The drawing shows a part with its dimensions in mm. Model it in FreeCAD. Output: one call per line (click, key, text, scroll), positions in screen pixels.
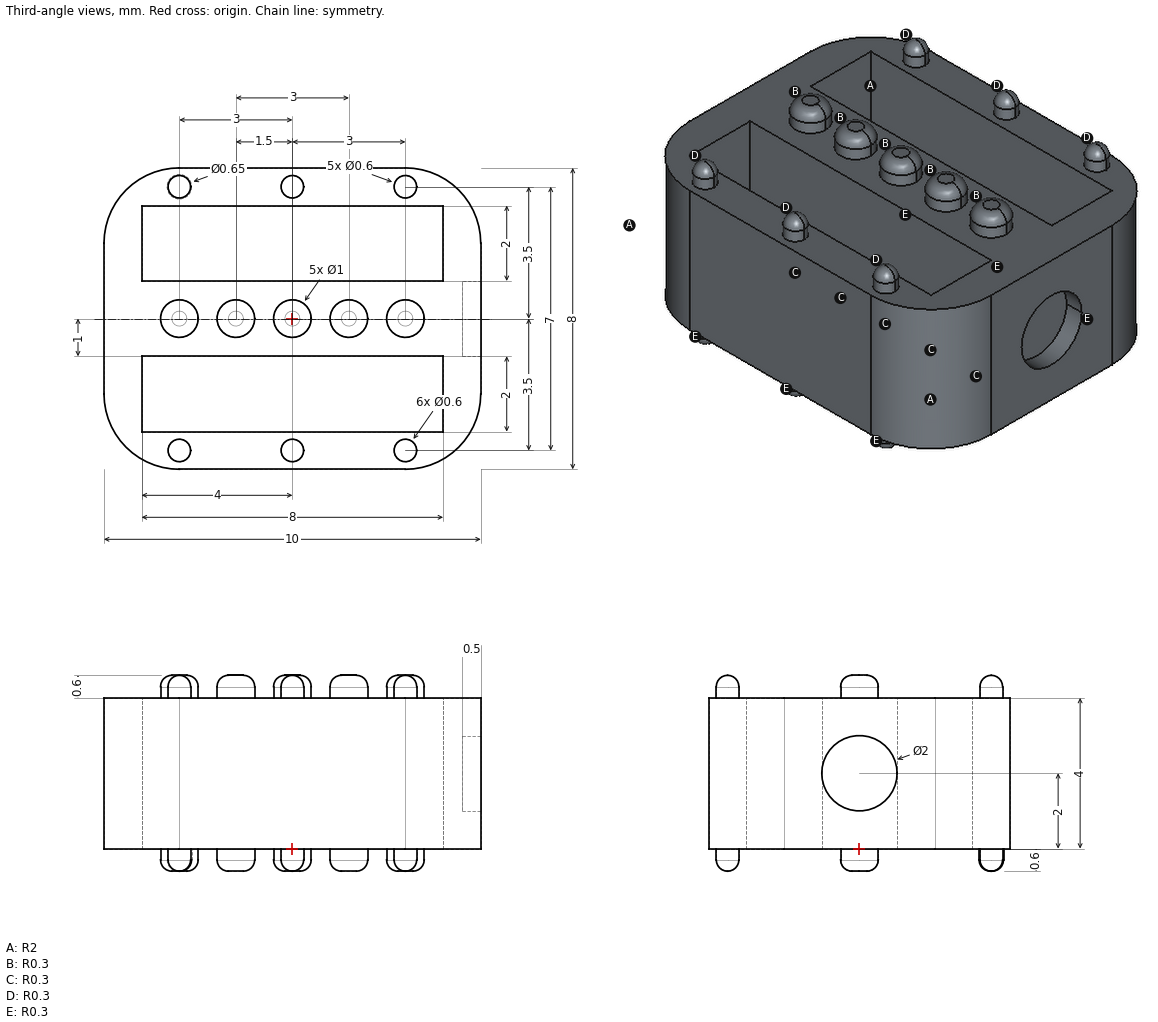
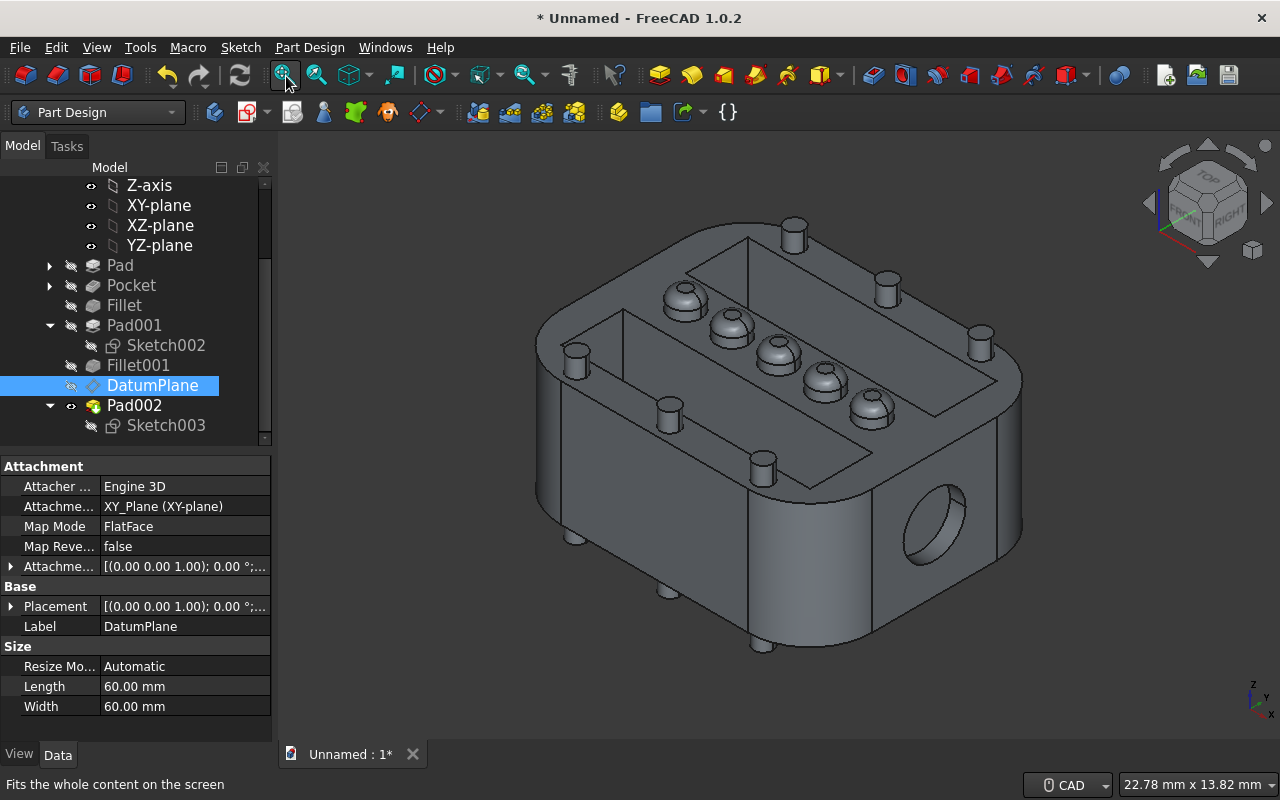
key(1)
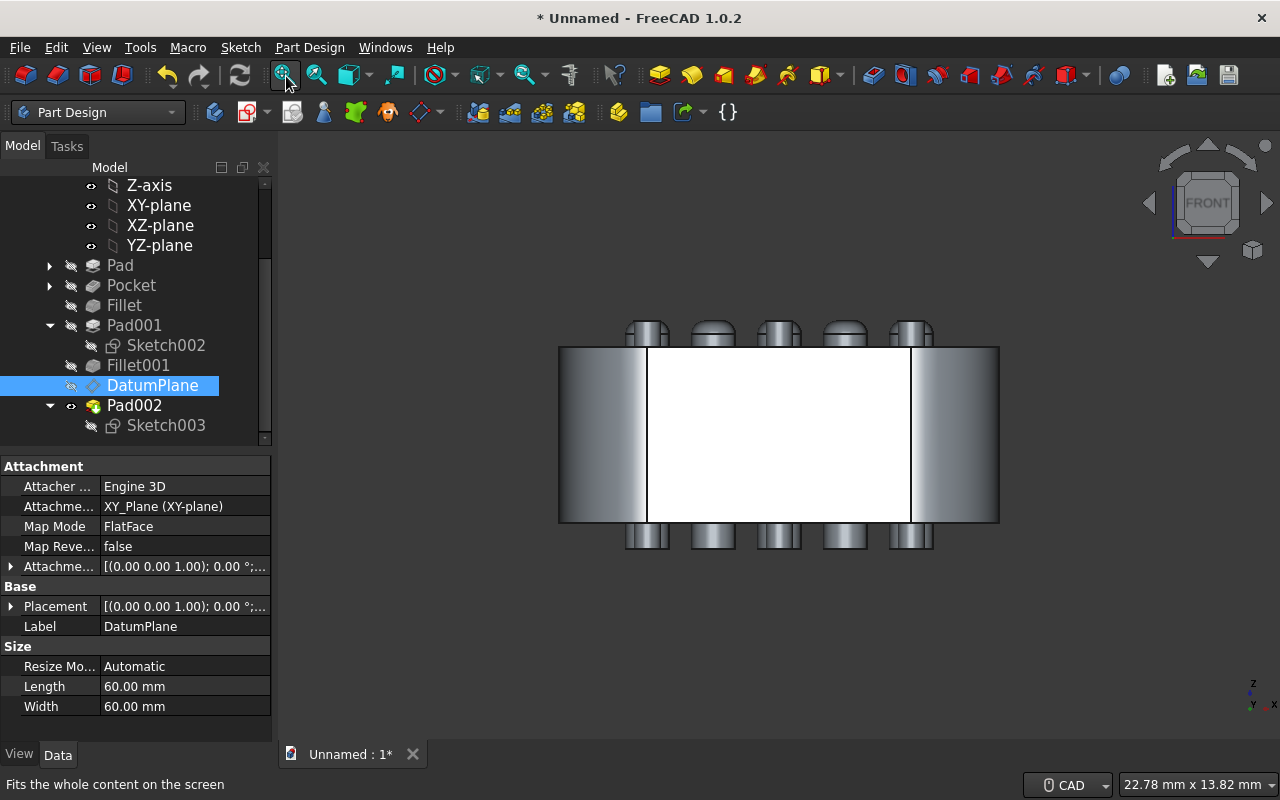
click(286, 76)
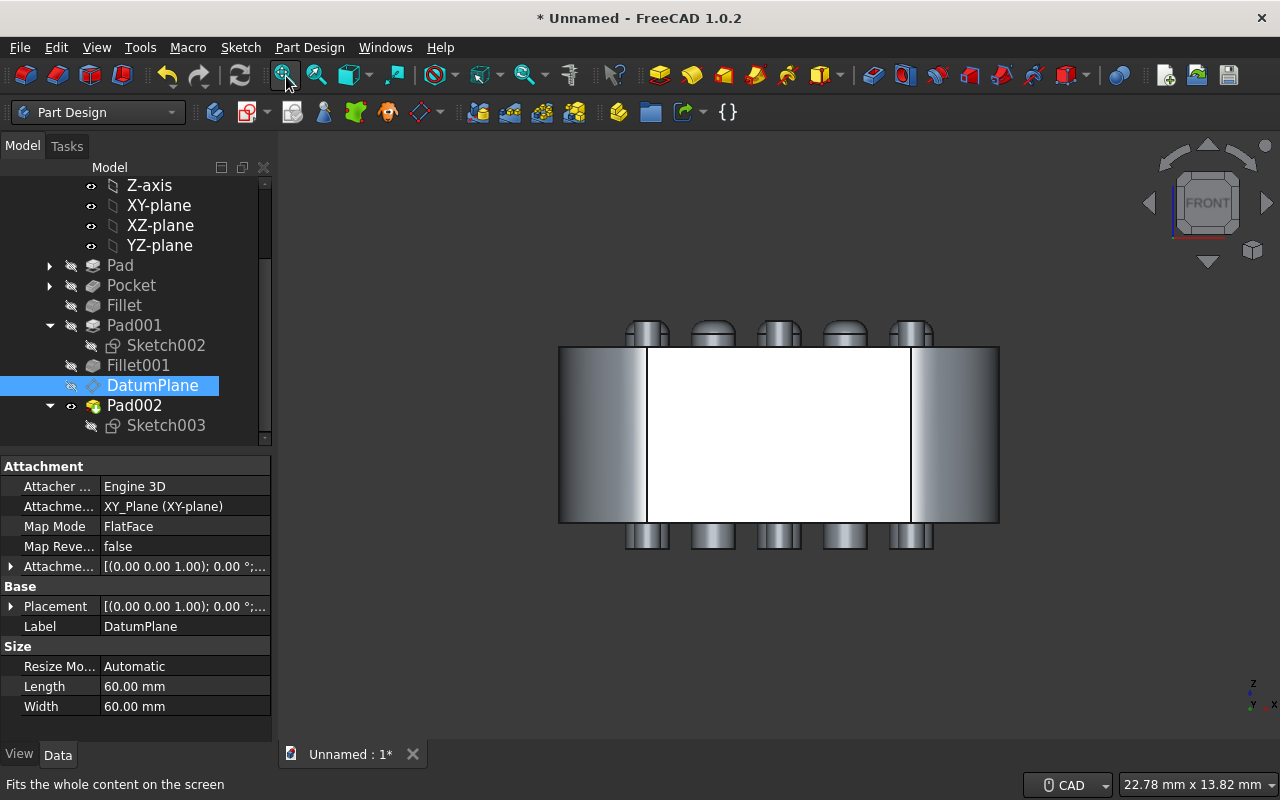
click(757, 548)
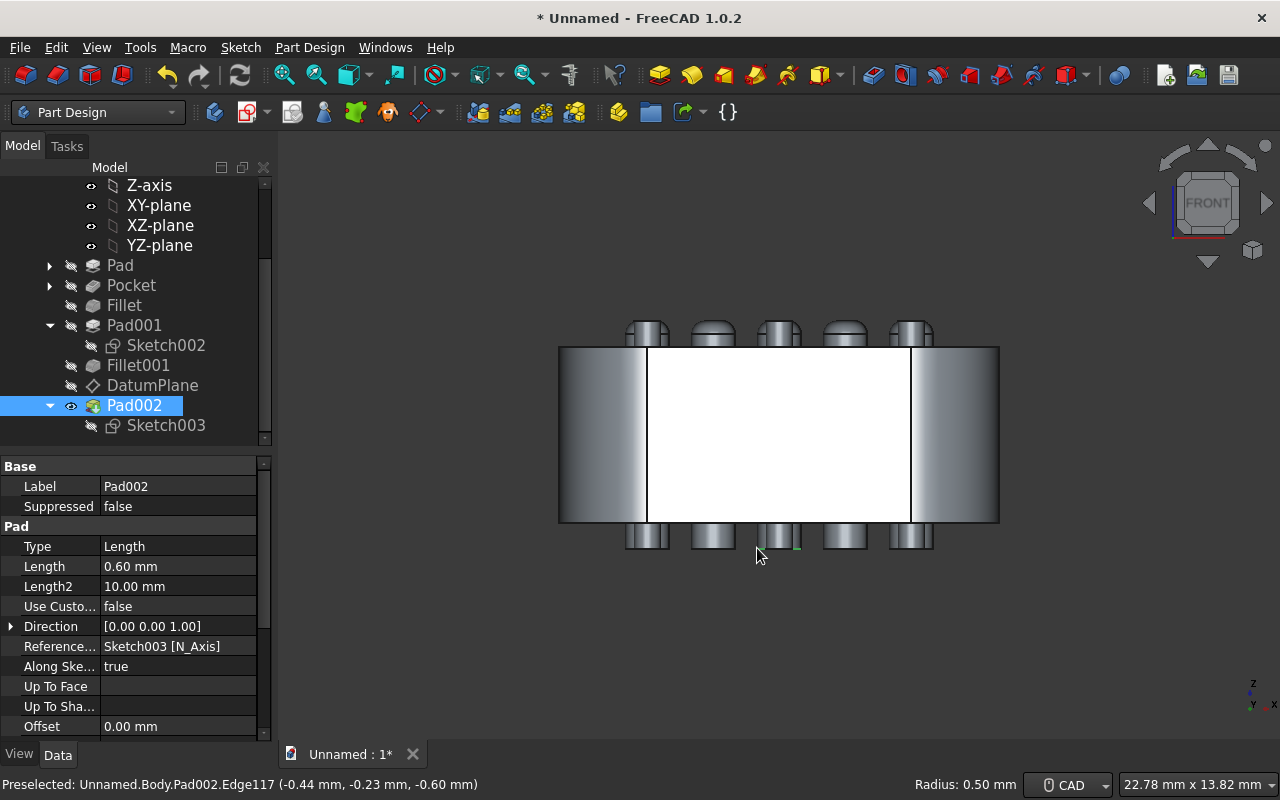
click(691, 548, ctrl)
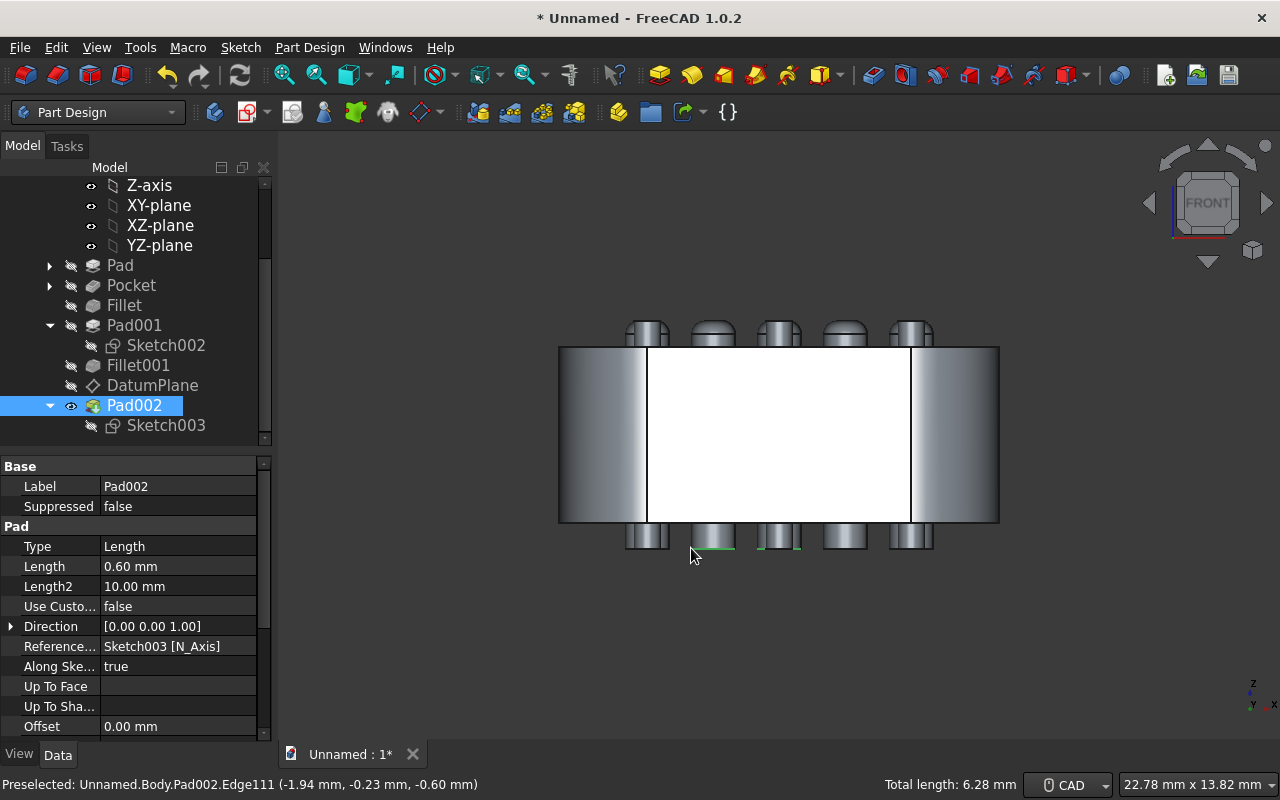
click(625, 548, ctrl)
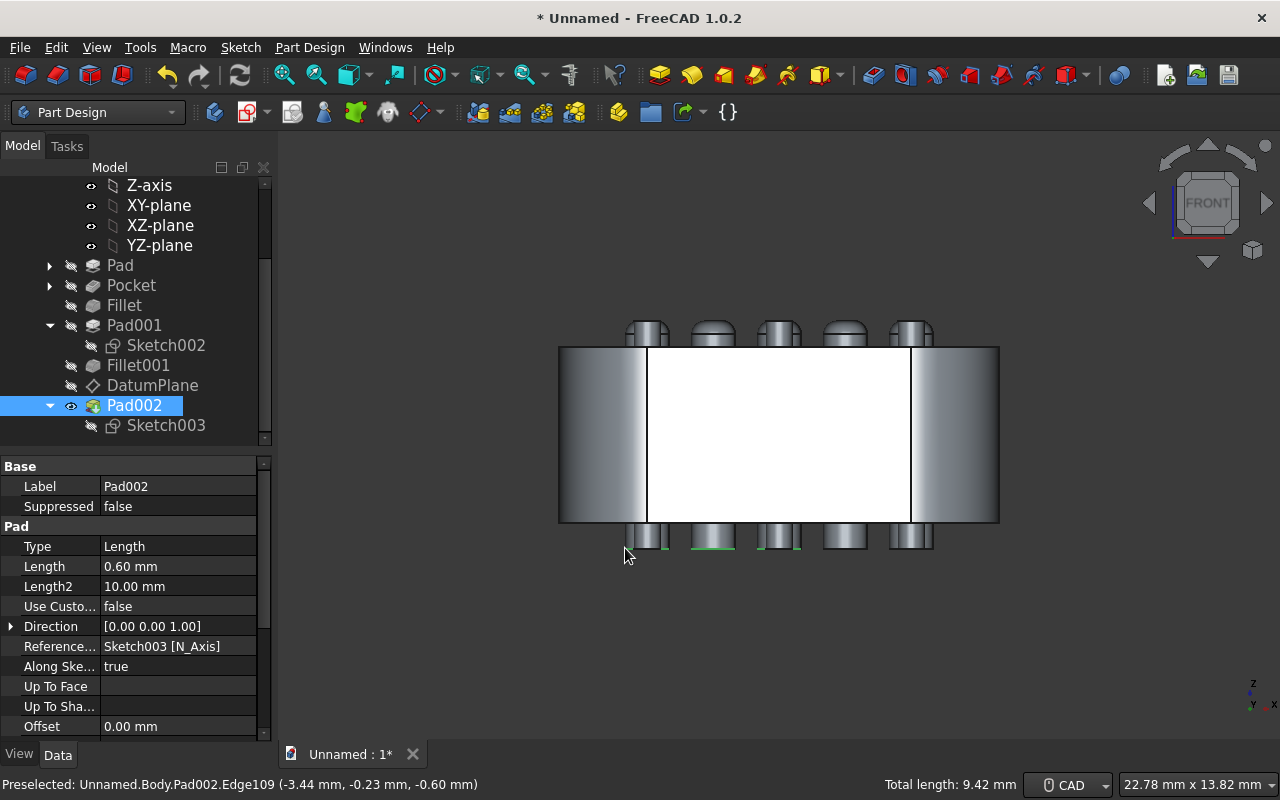
click(823, 548, ctrl)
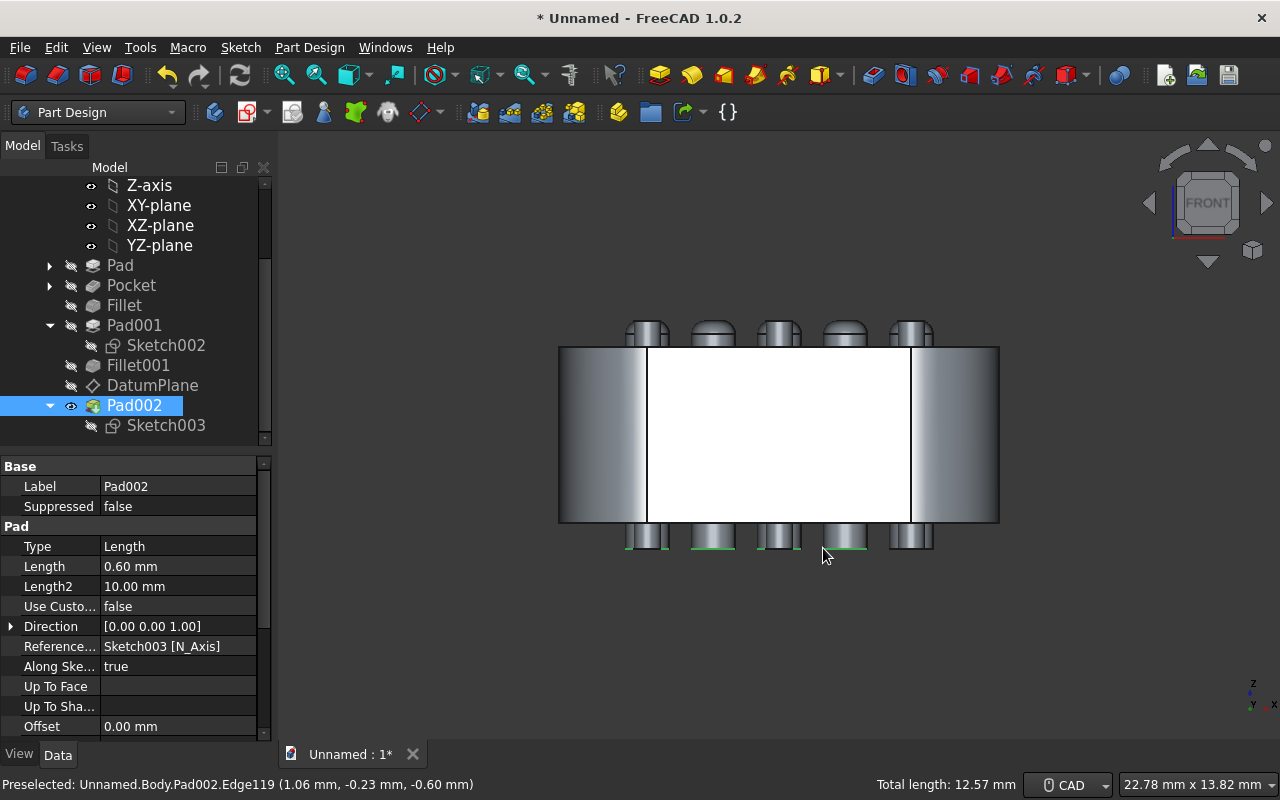
click(889, 548, ctrl)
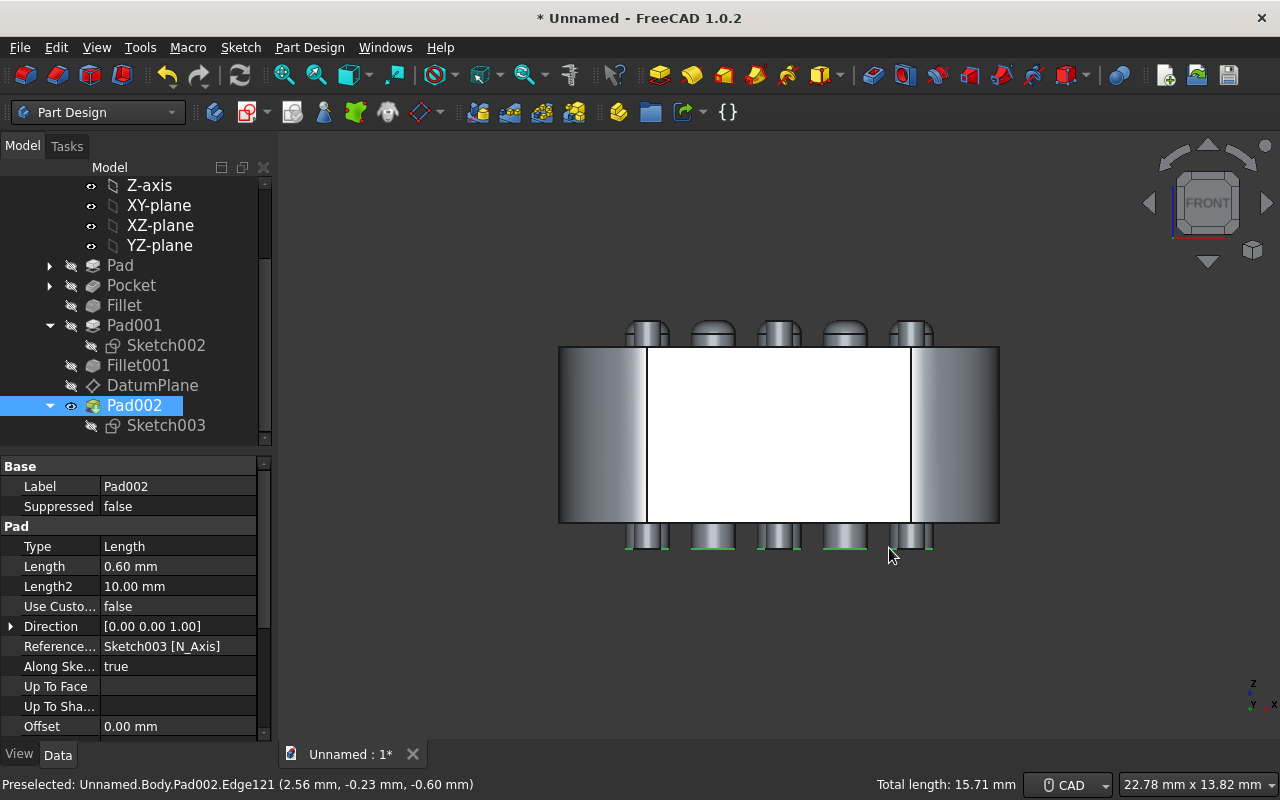
click(26, 76)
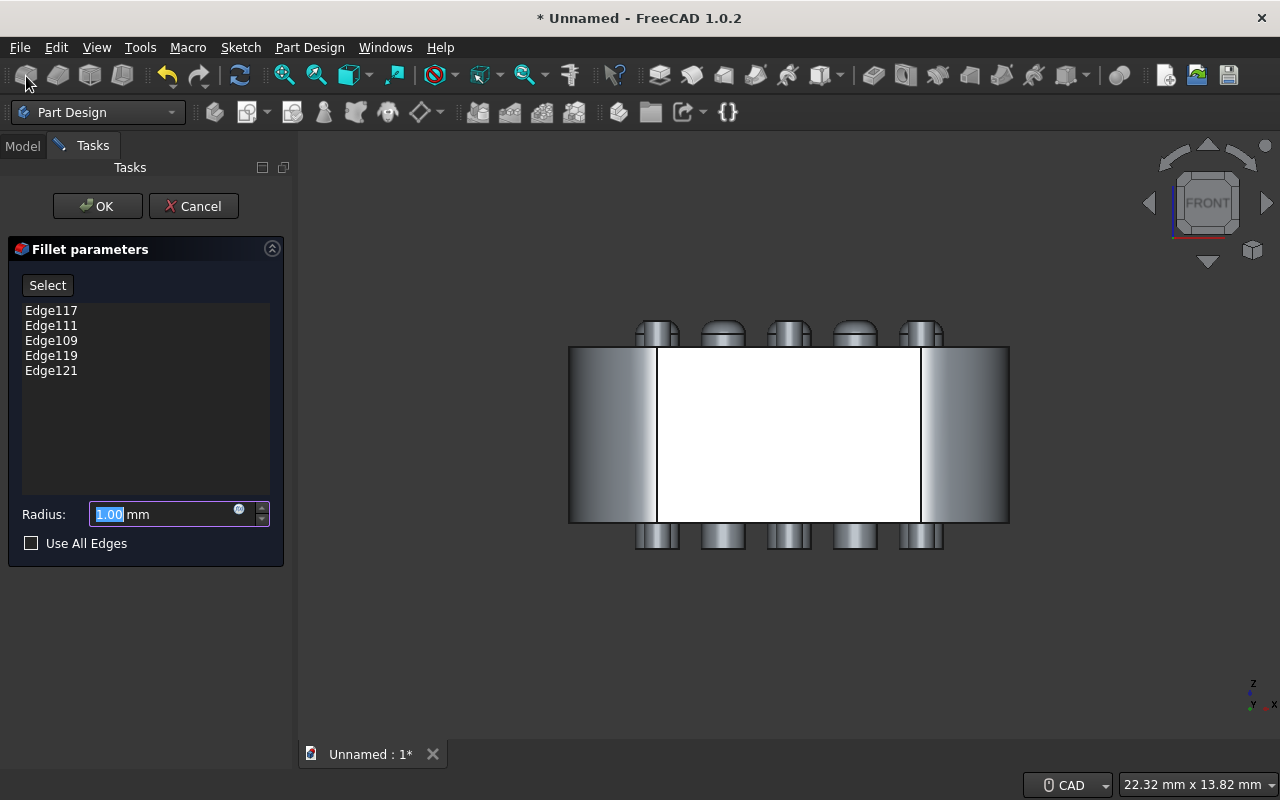
text(0.3)
key(Tab)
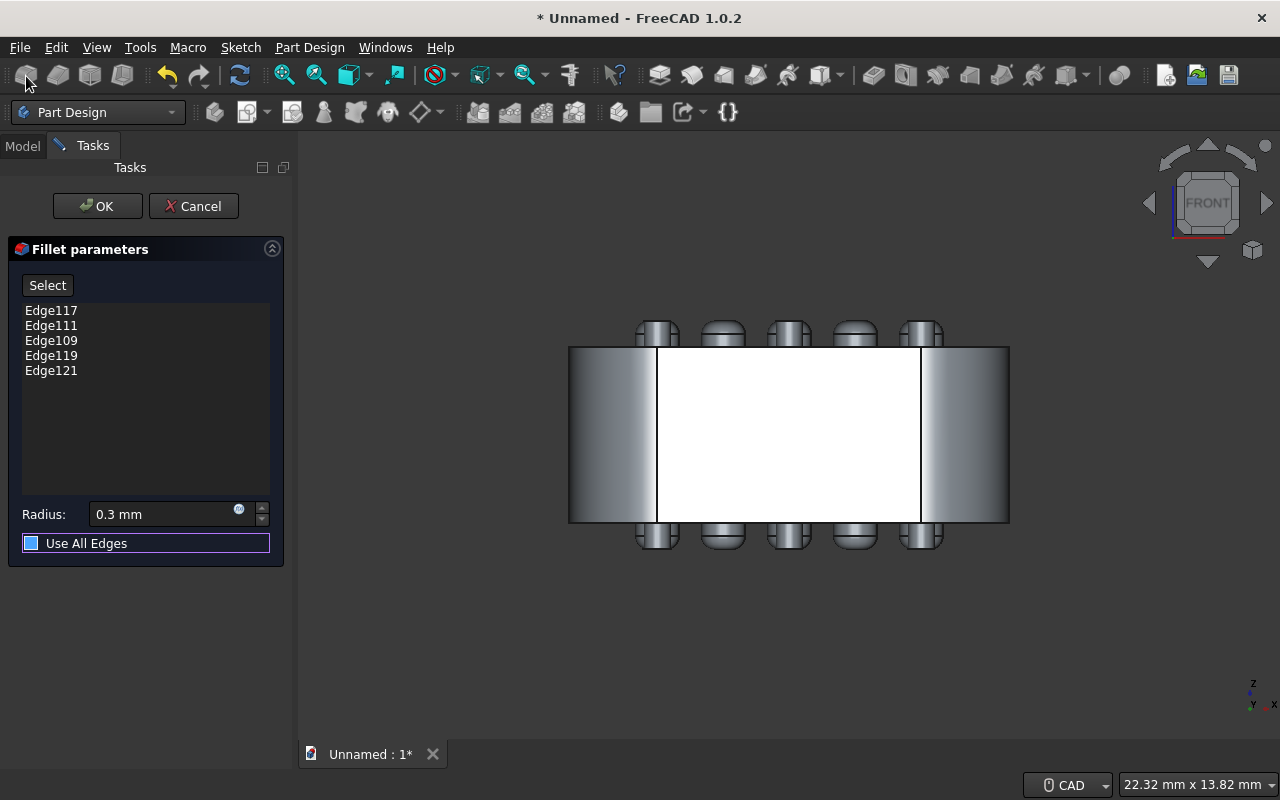
click(98, 206)